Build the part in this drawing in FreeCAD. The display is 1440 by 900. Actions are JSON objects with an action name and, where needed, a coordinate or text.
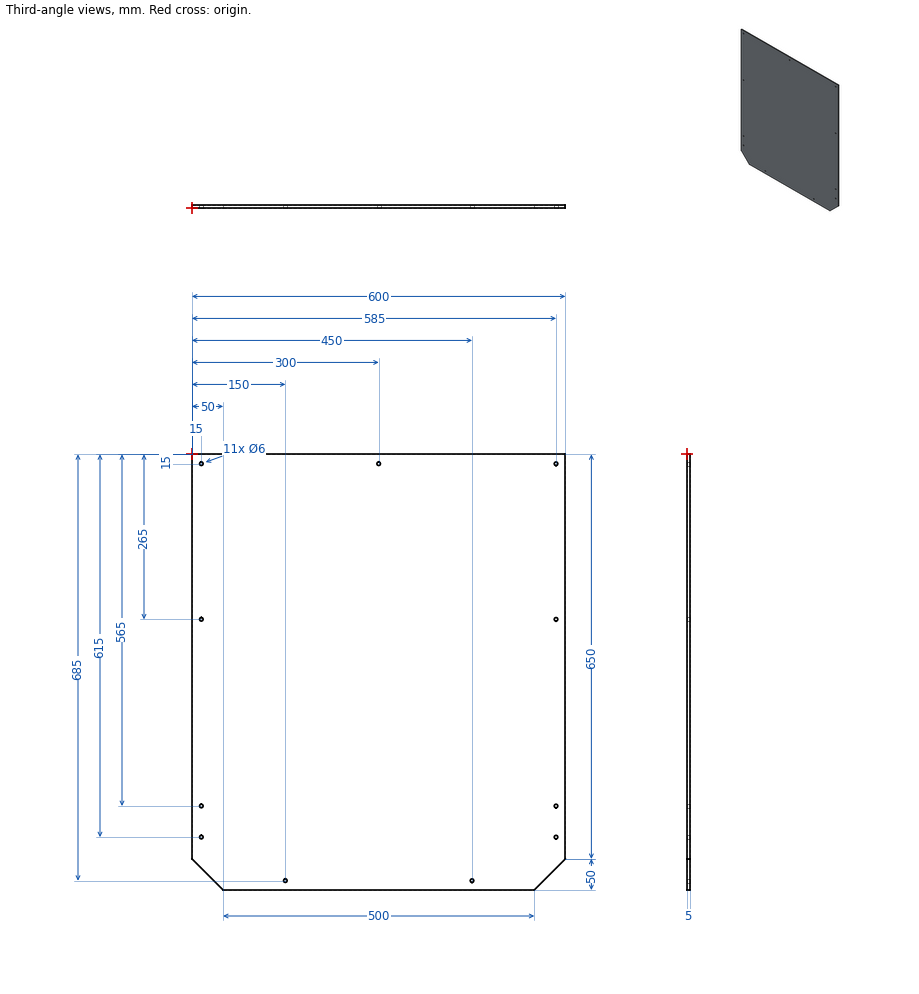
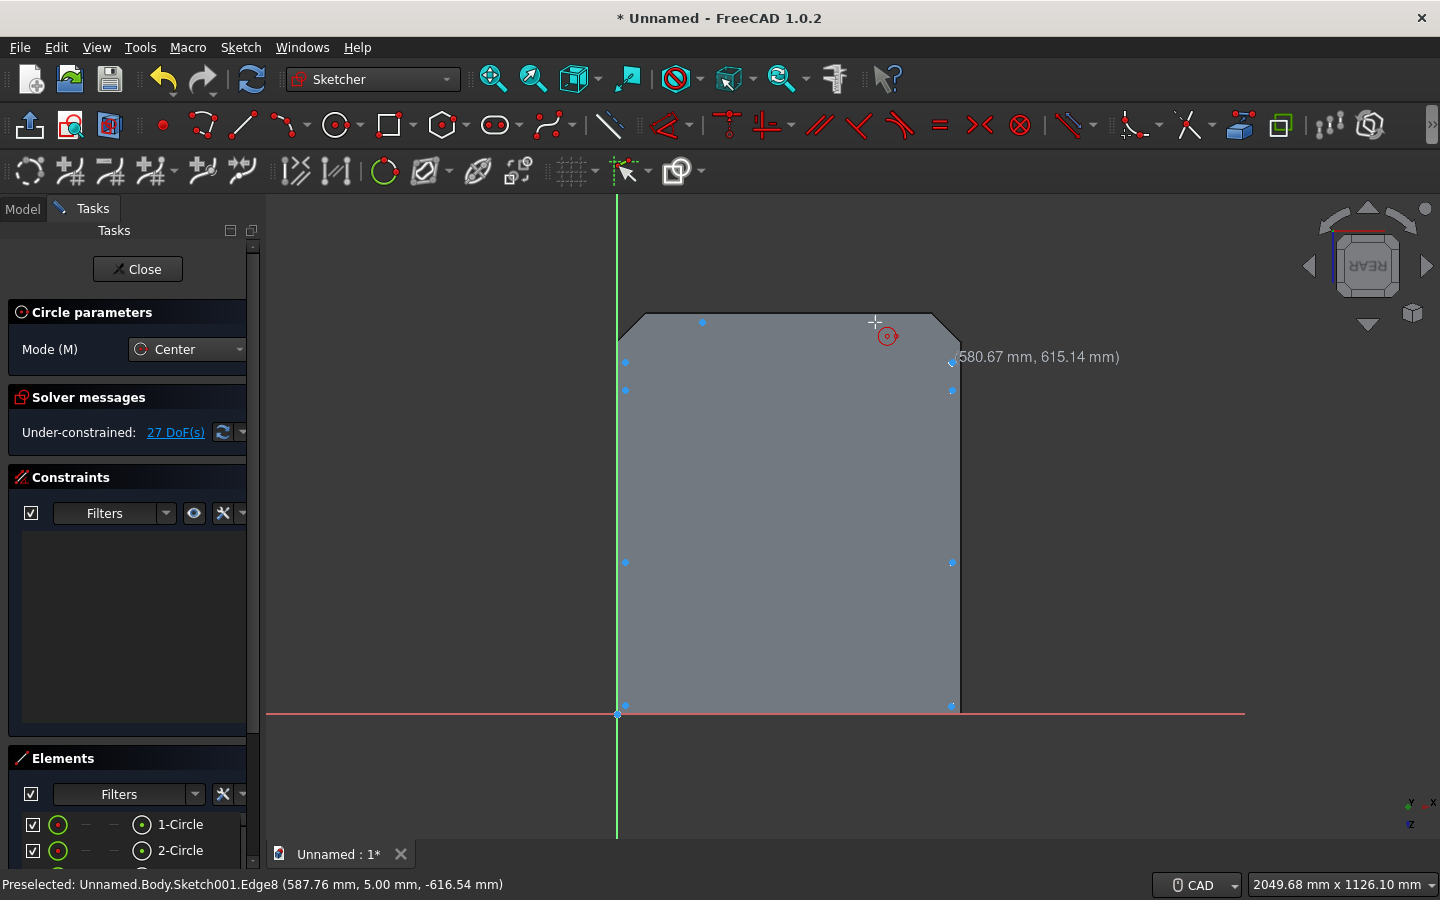
{"action": "left_click", "coordinate": [875, 322]}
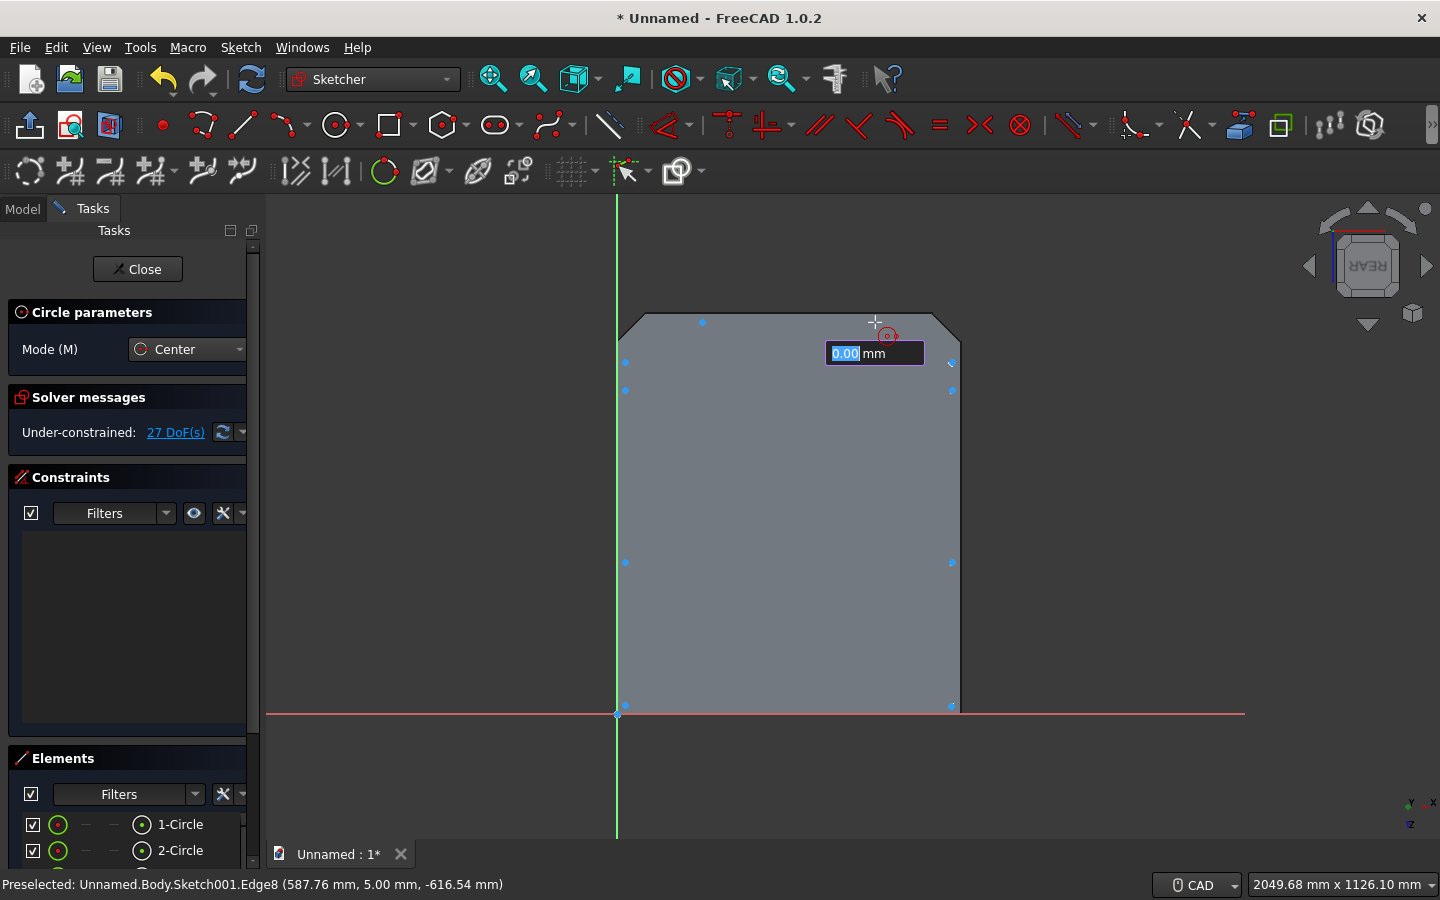
{"action": "scroll", "coordinate": [876, 321], "scroll_direction": "up", "scroll_amount": 12}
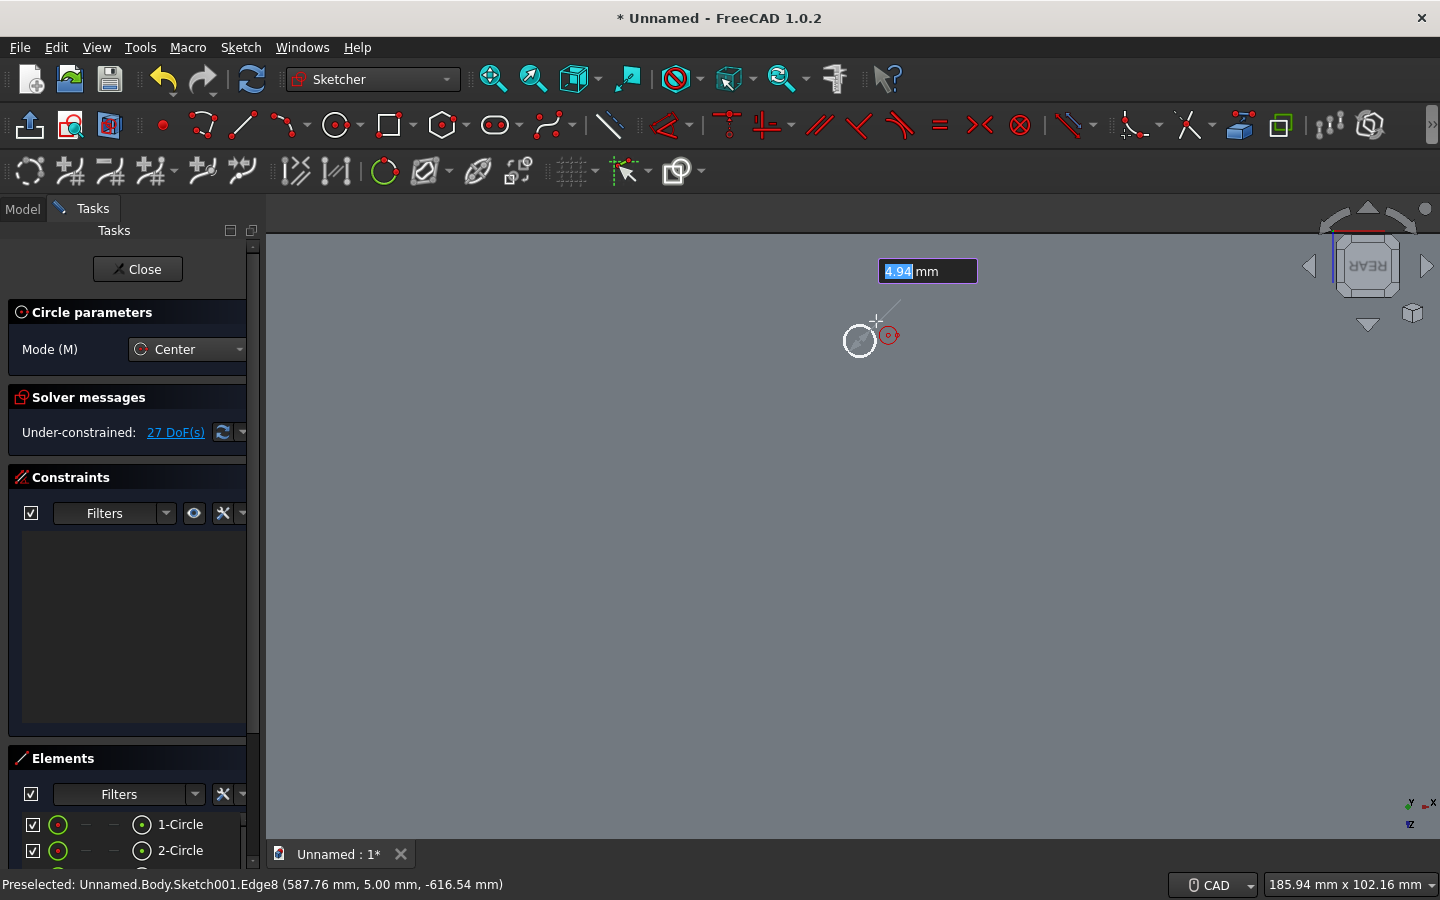
{"action": "left_click", "coordinate": [871, 314]}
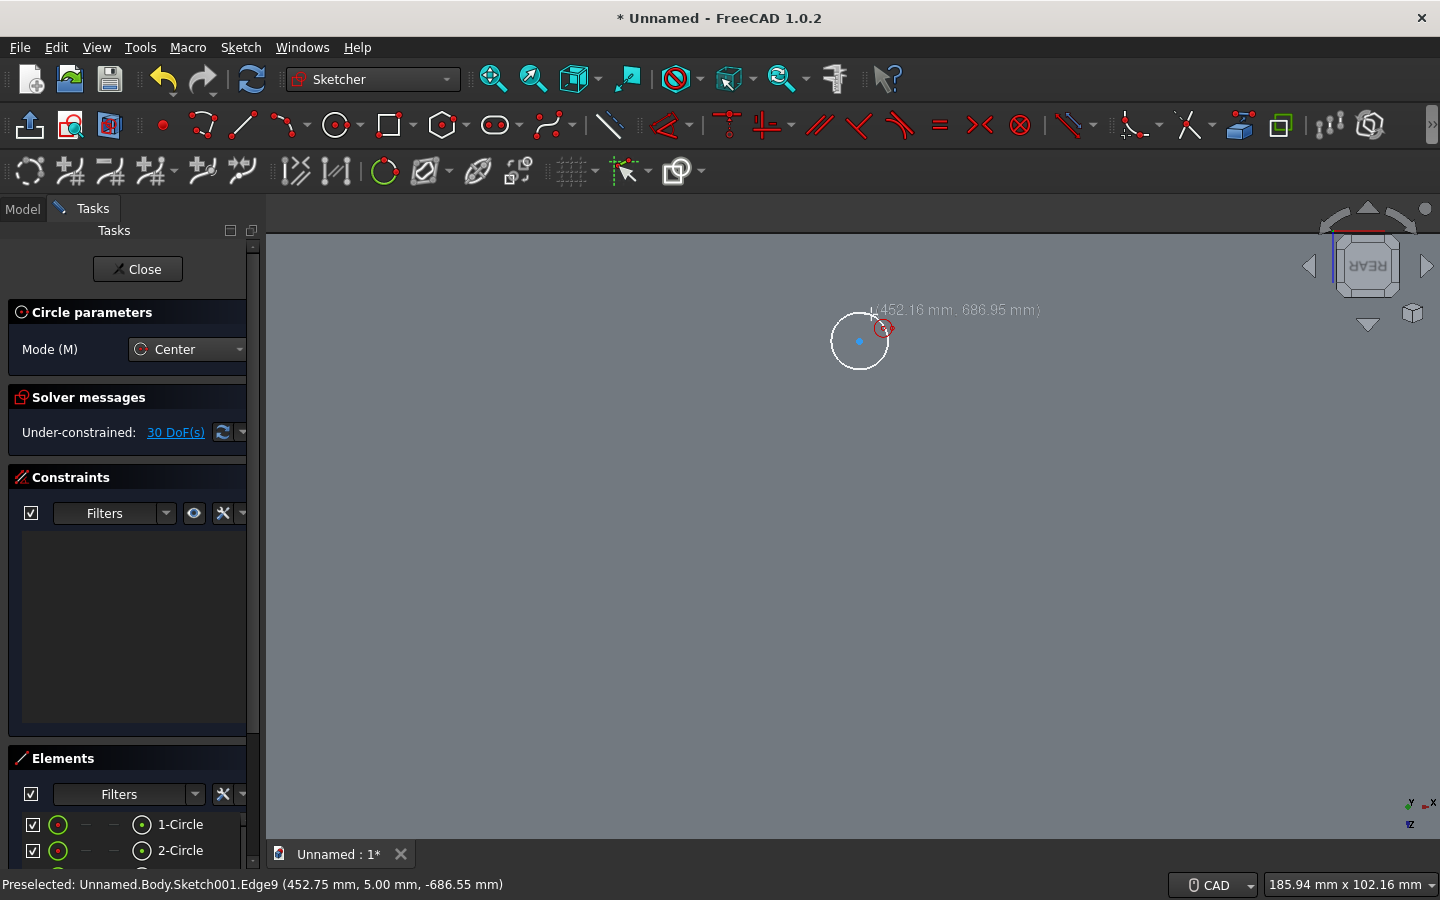
{"action": "scroll", "coordinate": [875, 321], "scroll_direction": "down", "scroll_amount": 12}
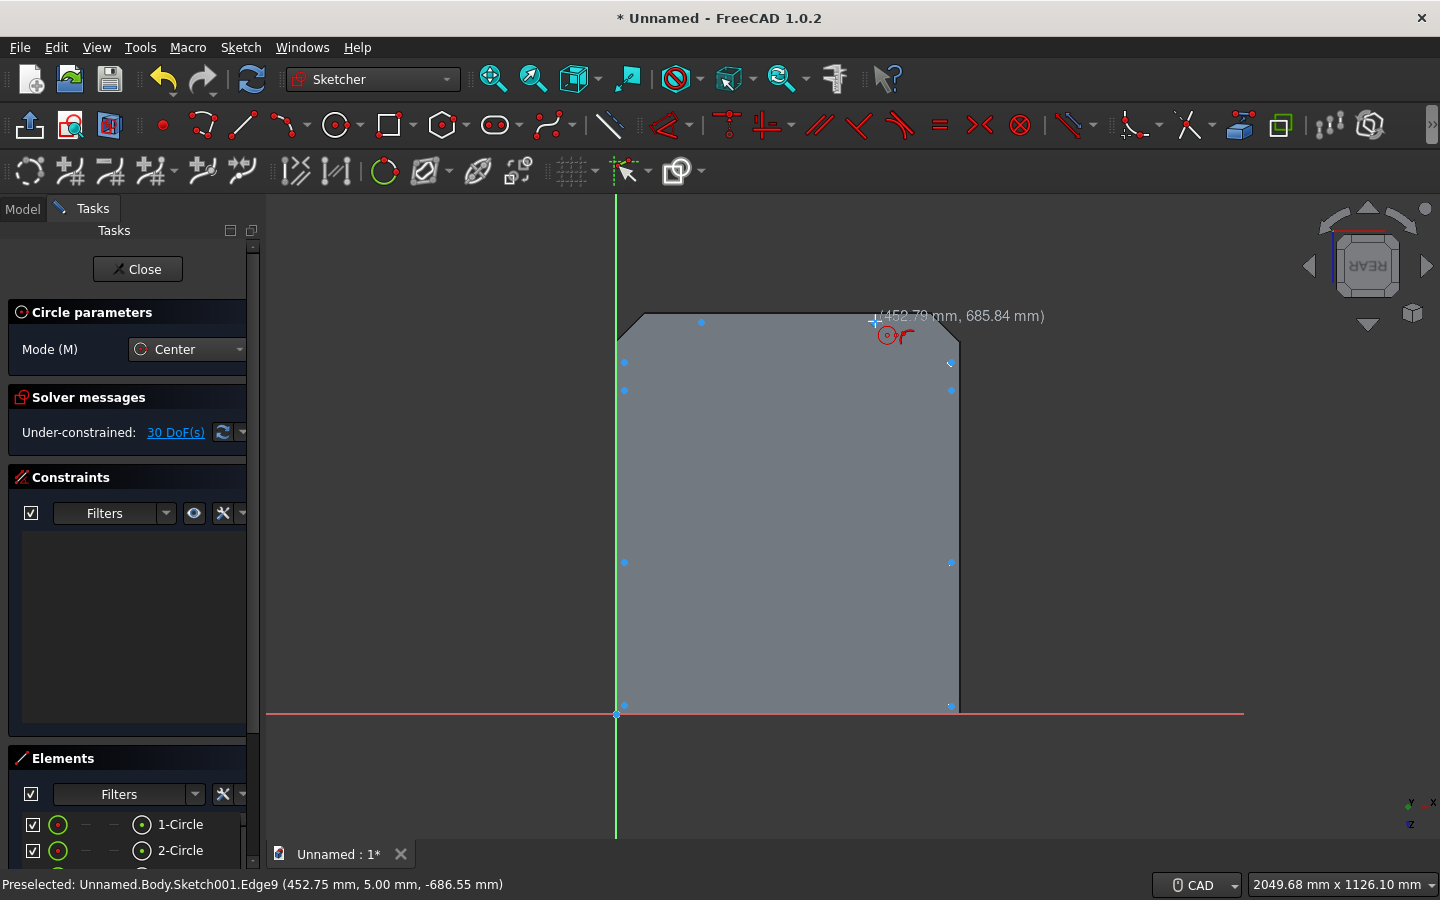
{"action": "scroll", "coordinate": [788, 706], "scroll_direction": "up", "scroll_amount": 13}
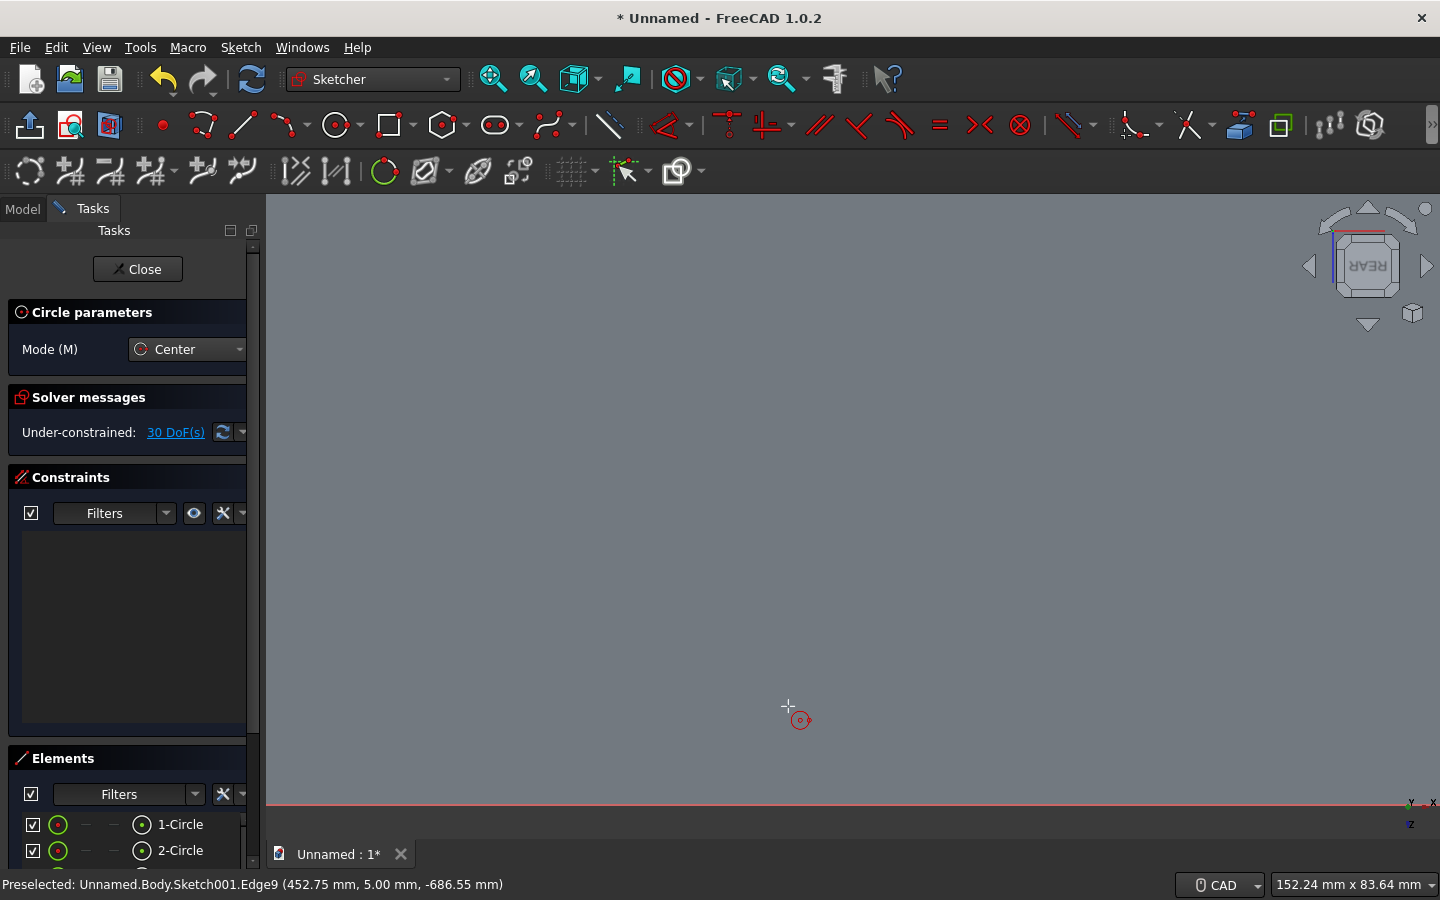
{"action": "scroll", "coordinate": [788, 706], "scroll_direction": "down", "scroll_amount": 13}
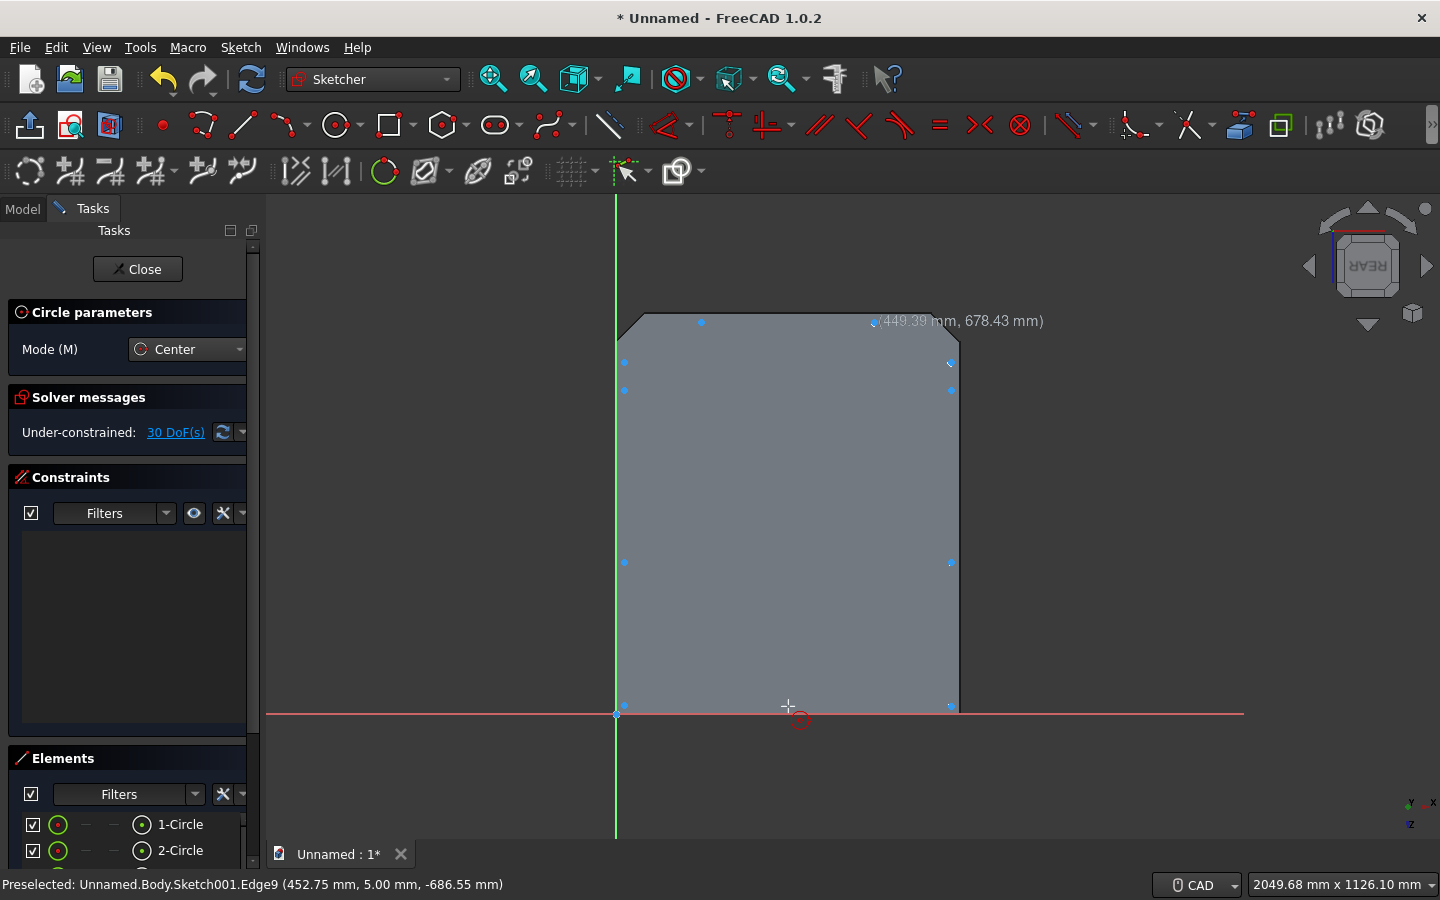
{"action": "scroll", "coordinate": [788, 706], "scroll_direction": "up", "scroll_amount": 4}